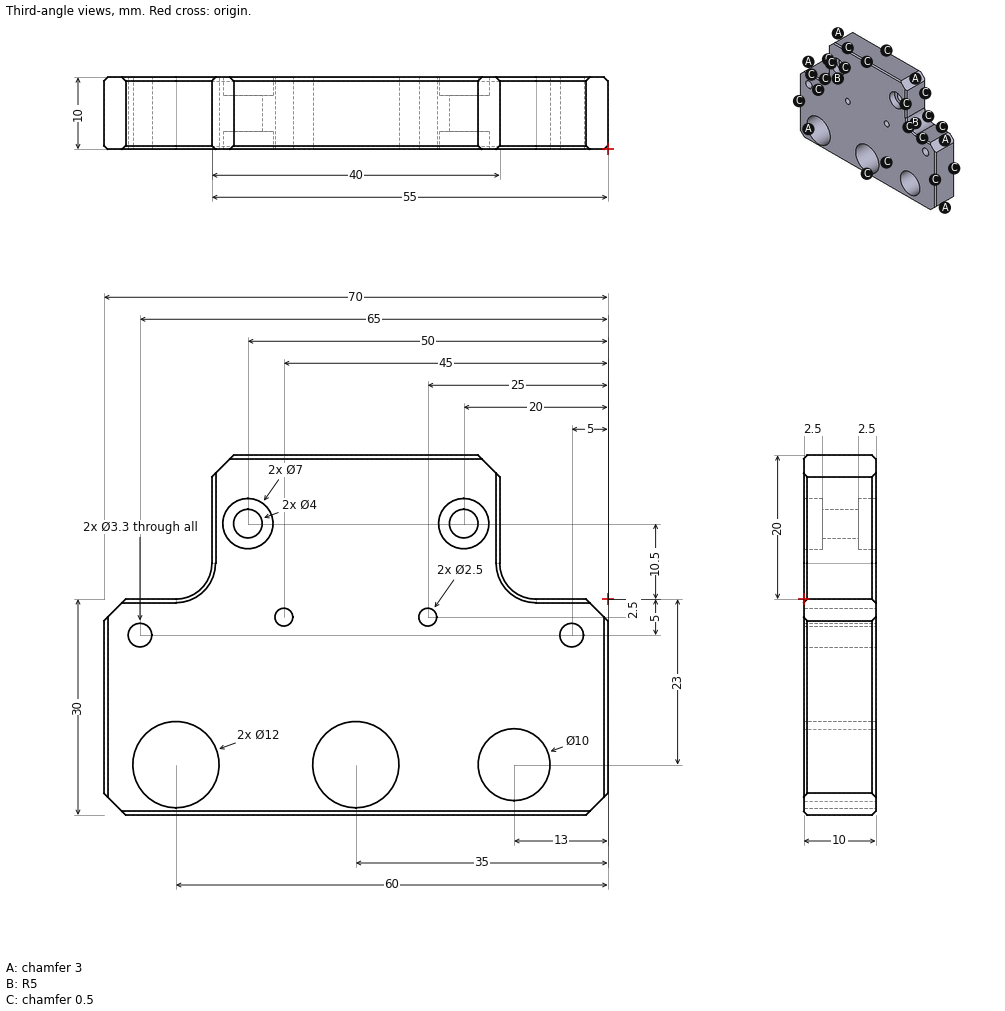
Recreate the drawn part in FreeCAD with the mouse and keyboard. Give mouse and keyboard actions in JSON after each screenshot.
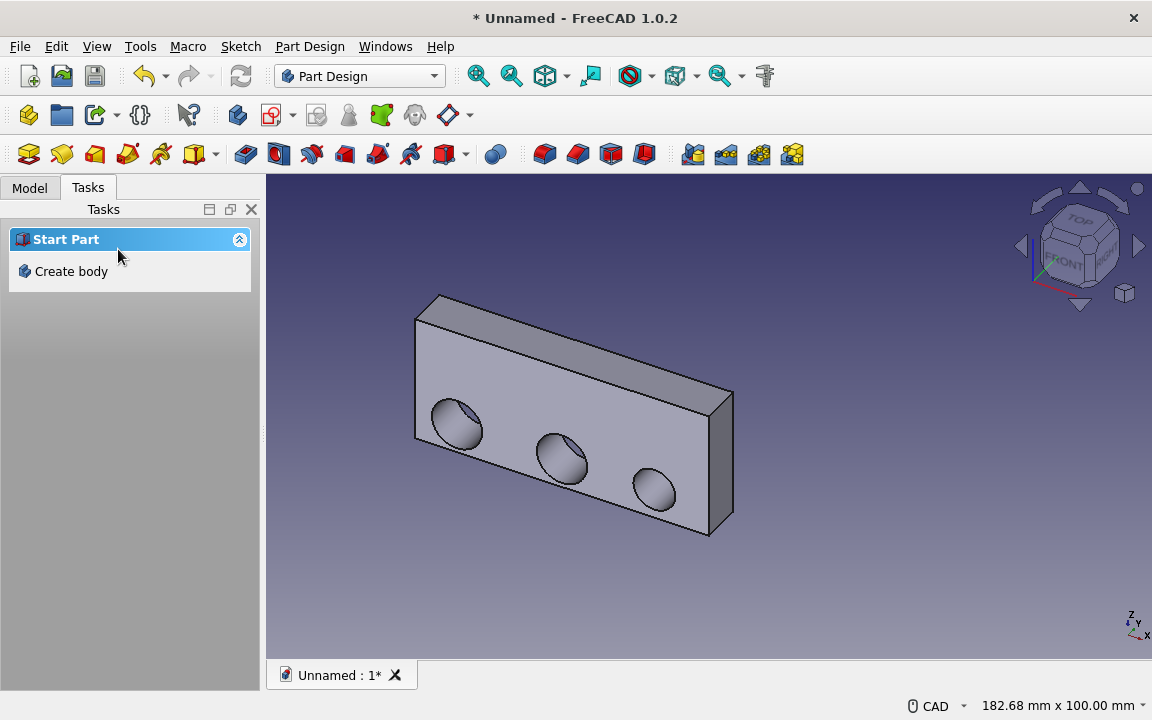
{"action": "left_click", "coordinate": [520, 395]}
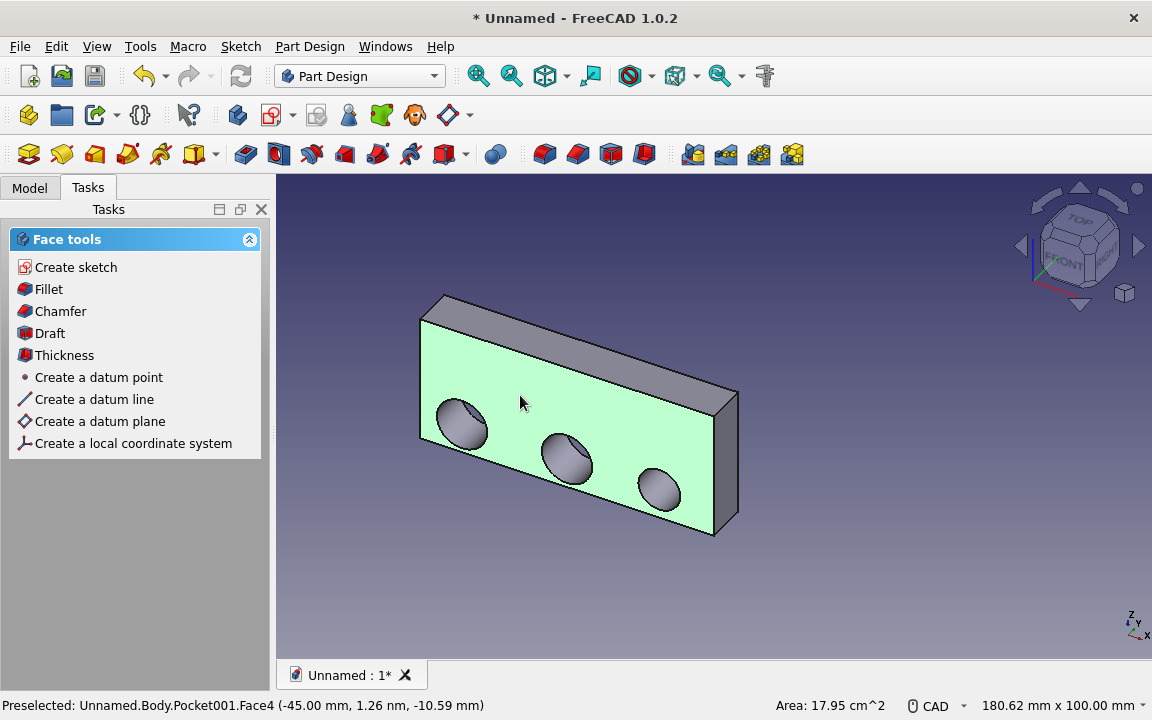
{"action": "left_click", "coordinate": [270, 116]}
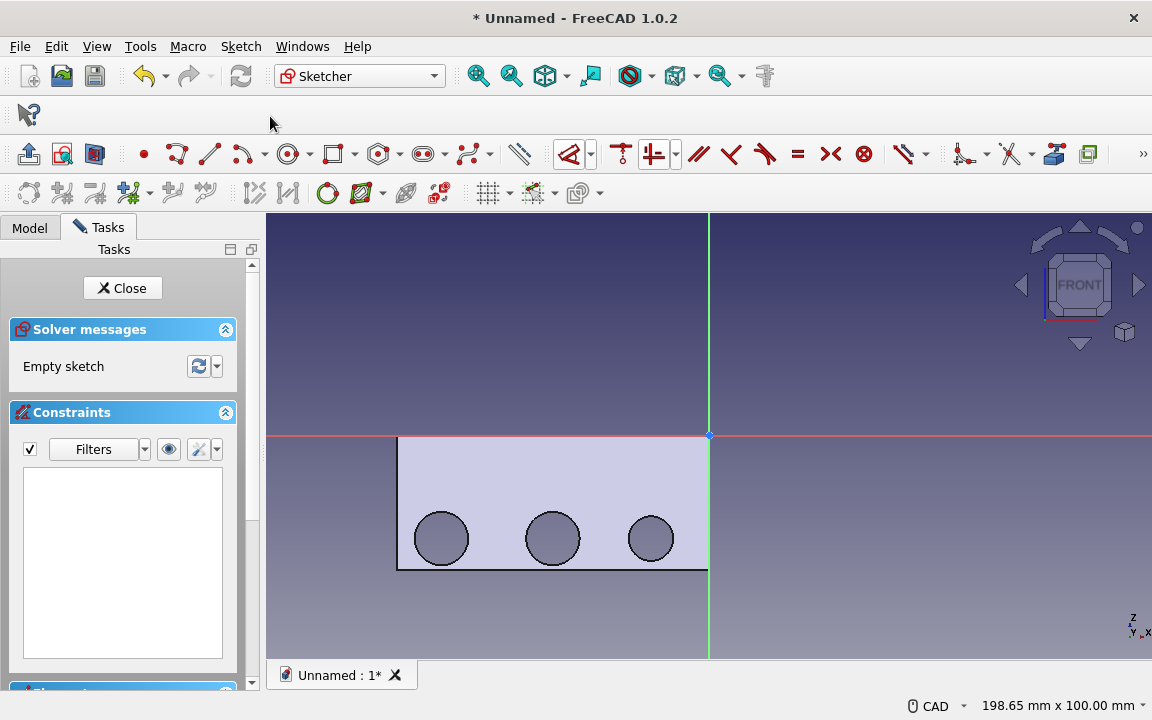
{"action": "scroll", "coordinate": [397, 481], "scroll_direction": "up", "scroll_amount": 2}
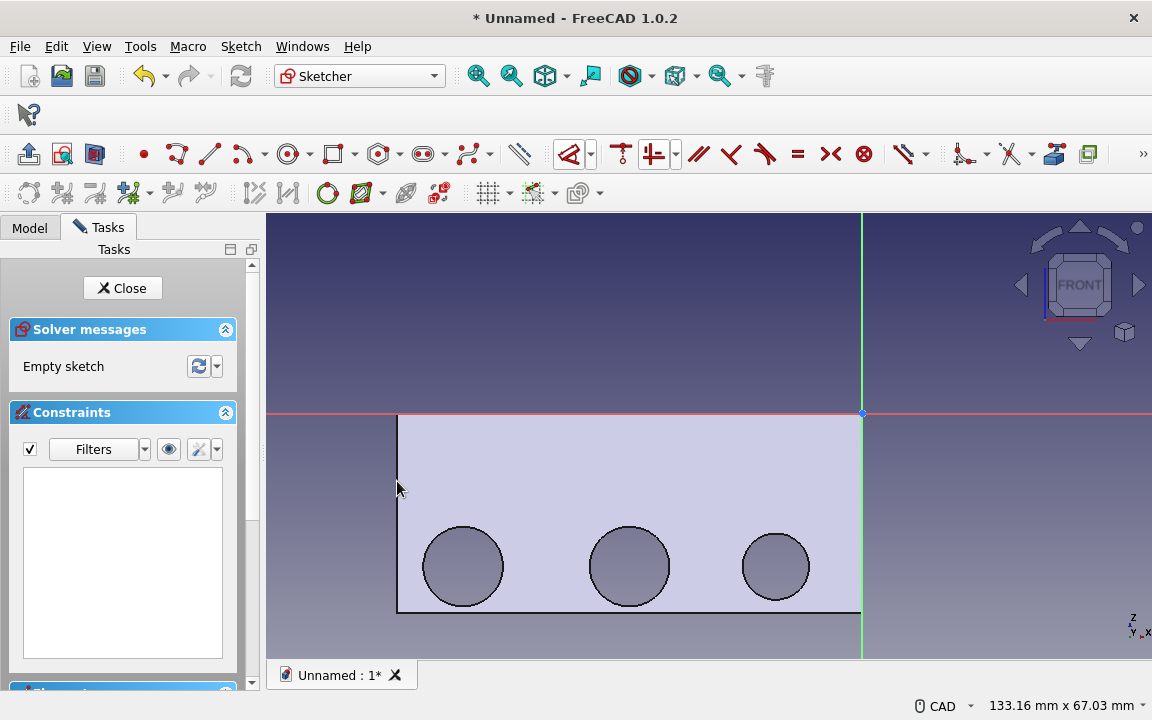
{"action": "left_click", "coordinate": [288, 154]}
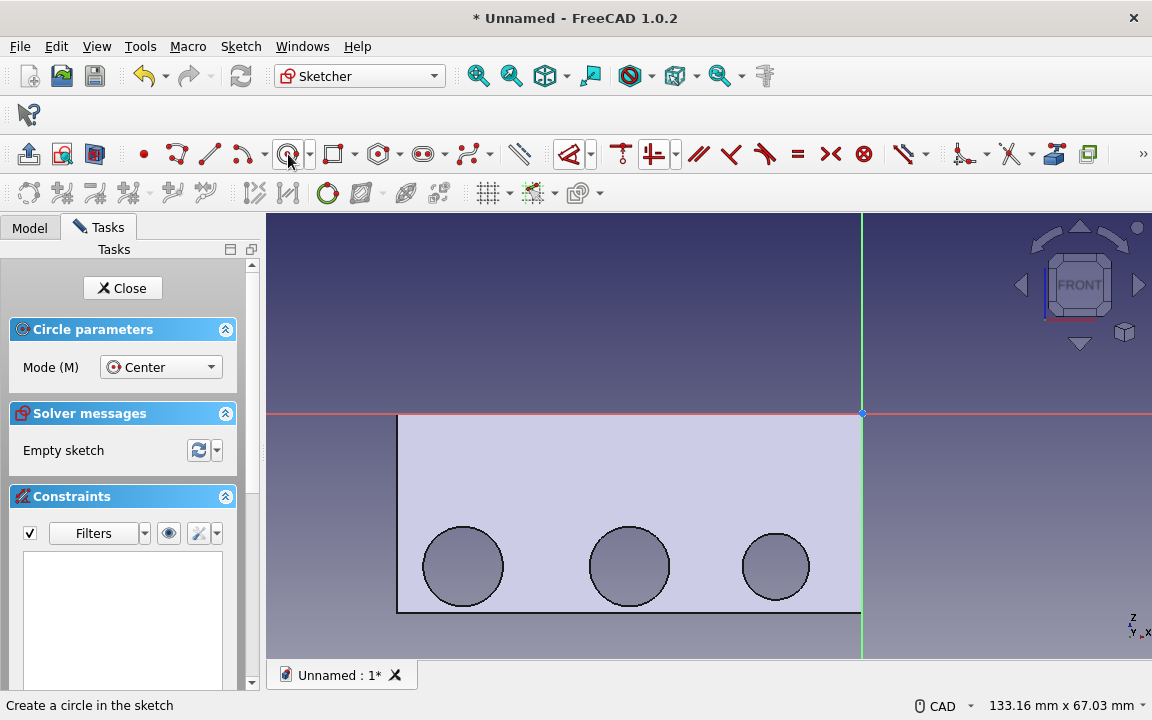
{"action": "scroll", "coordinate": [430, 447], "scroll_direction": "up", "scroll_amount": 4}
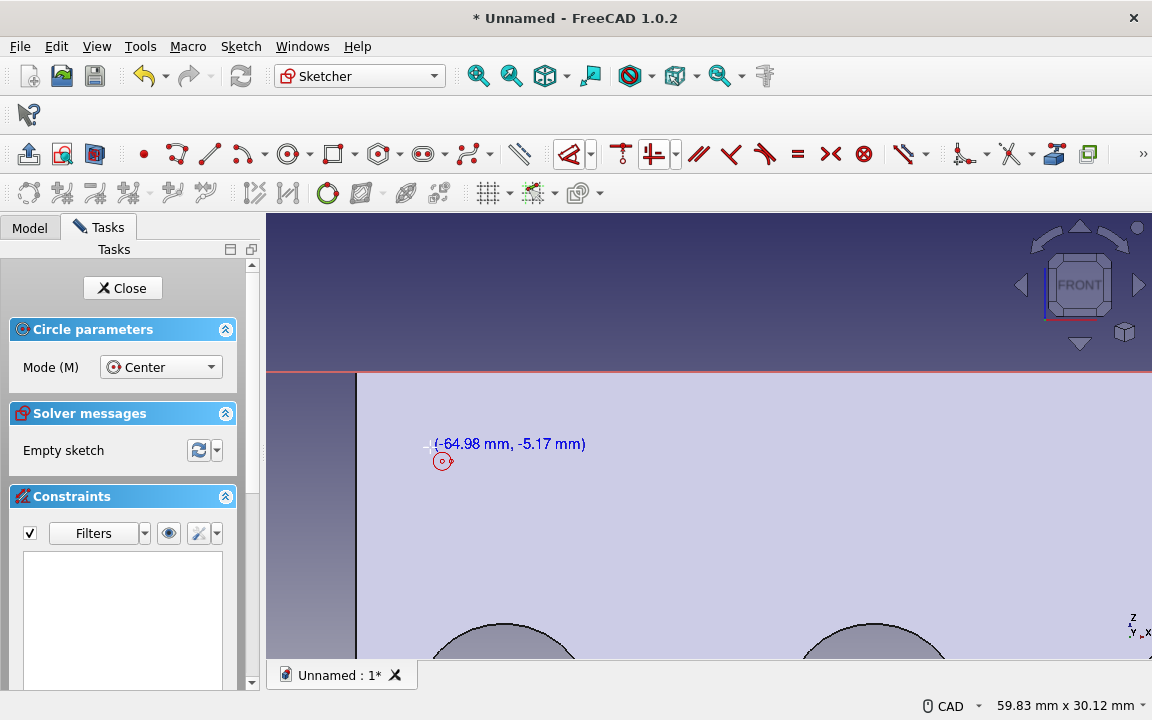
{"action": "left_click", "coordinate": [430, 446]}
{"action": "left_click", "coordinate": [447, 429]}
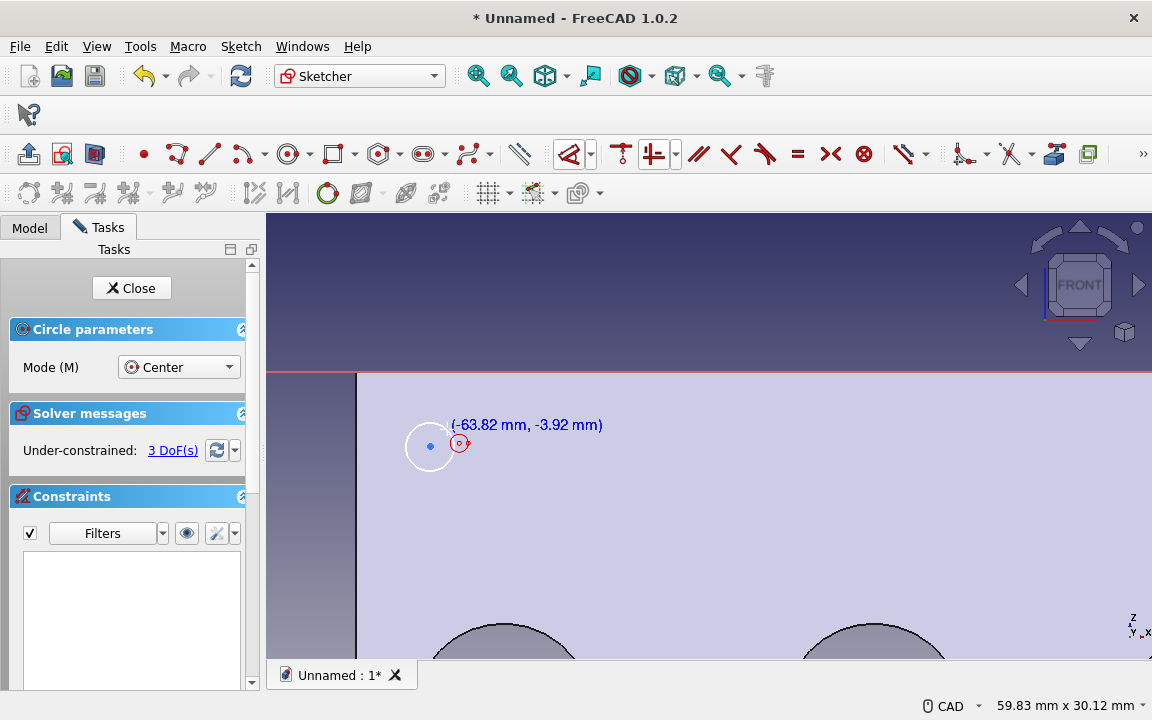
{"action": "scroll", "coordinate": [430, 448], "scroll_direction": "down", "scroll_amount": 4}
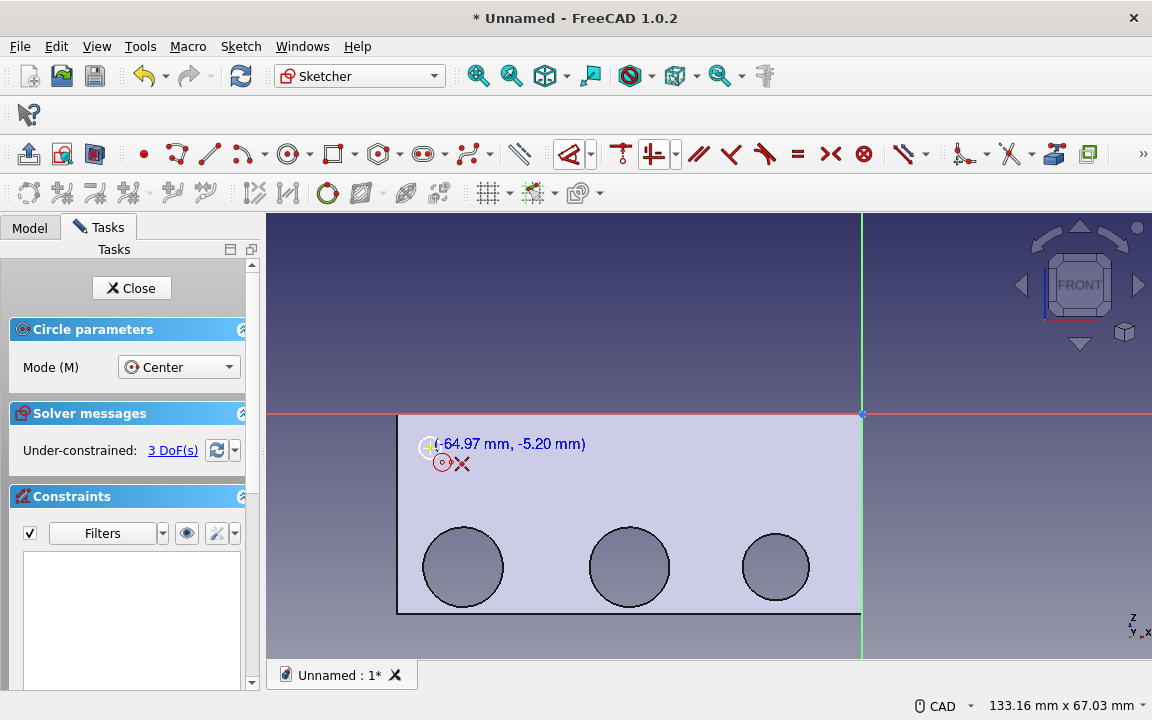
{"action": "scroll", "coordinate": [829, 447], "scroll_direction": "up", "scroll_amount": 4}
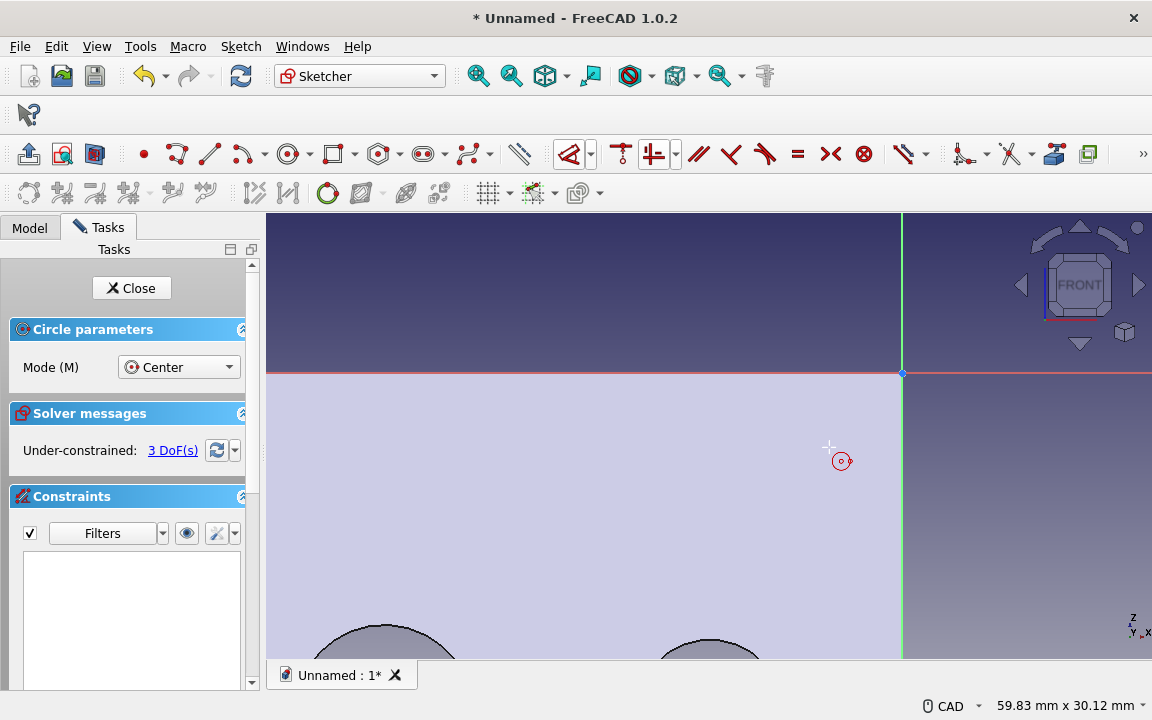
{"action": "left_click", "coordinate": [828, 447]}
{"action": "left_click", "coordinate": [846, 430]}
{"action": "key", "text": "Escape"}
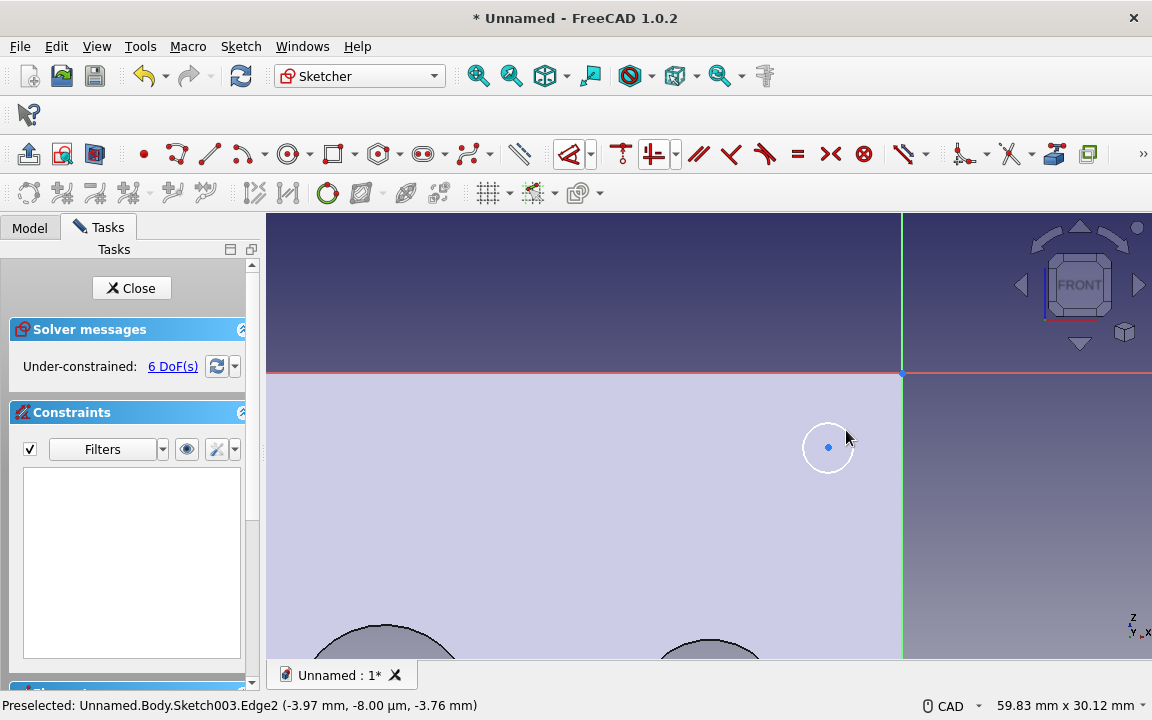
{"action": "scroll", "coordinate": [829, 447], "scroll_direction": "down", "scroll_amount": 4}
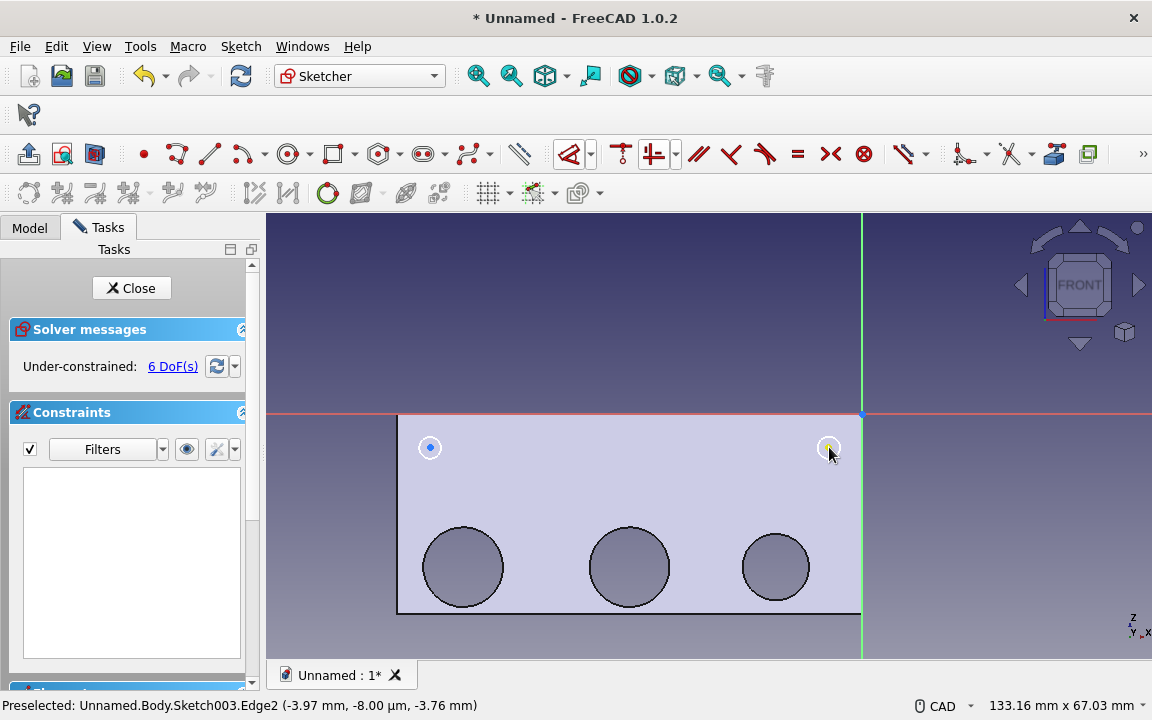
{"action": "scroll", "coordinate": [438, 440], "scroll_direction": "up", "scroll_amount": 2}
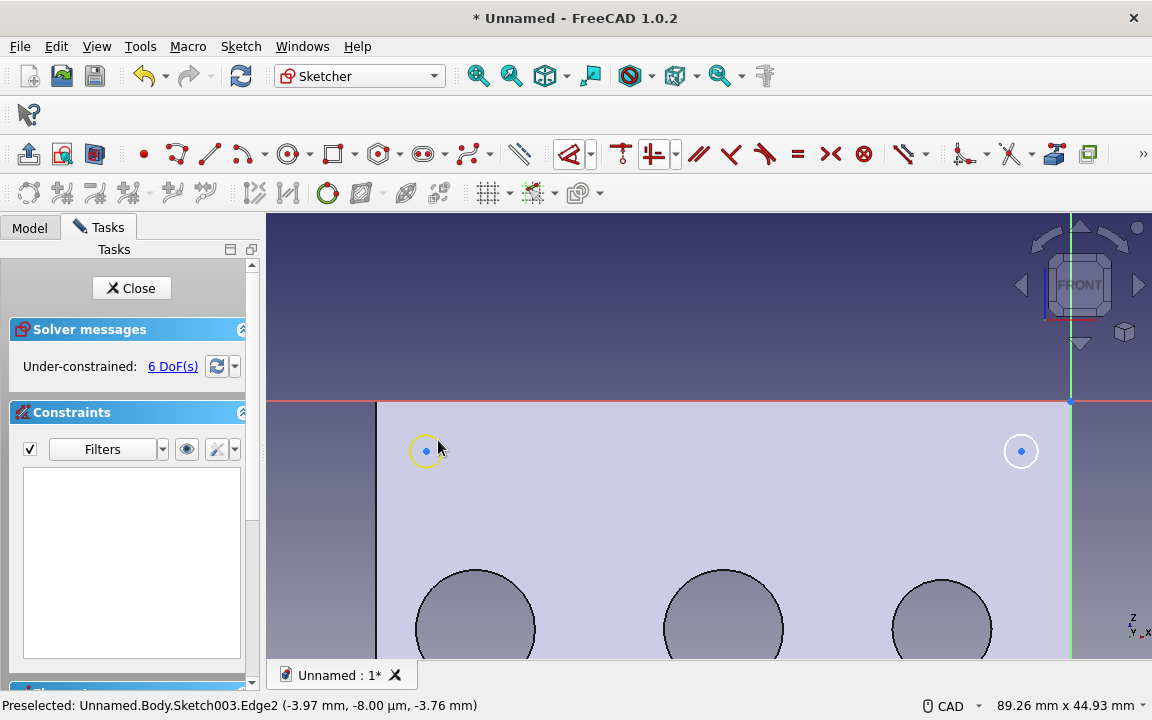
{"action": "left_click", "coordinate": [437, 440]}